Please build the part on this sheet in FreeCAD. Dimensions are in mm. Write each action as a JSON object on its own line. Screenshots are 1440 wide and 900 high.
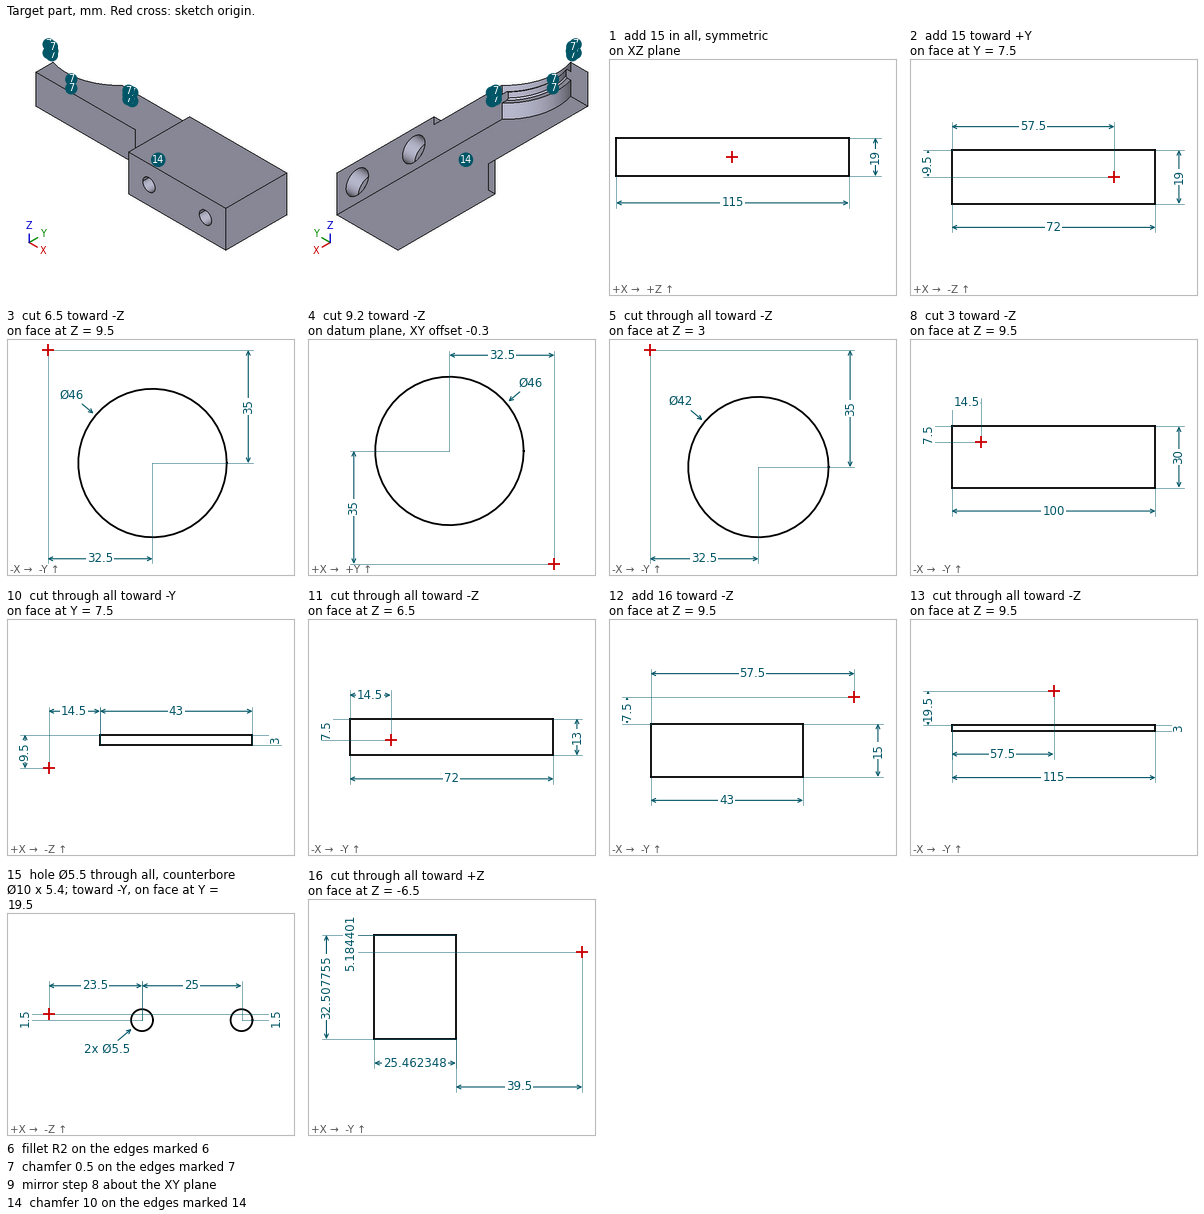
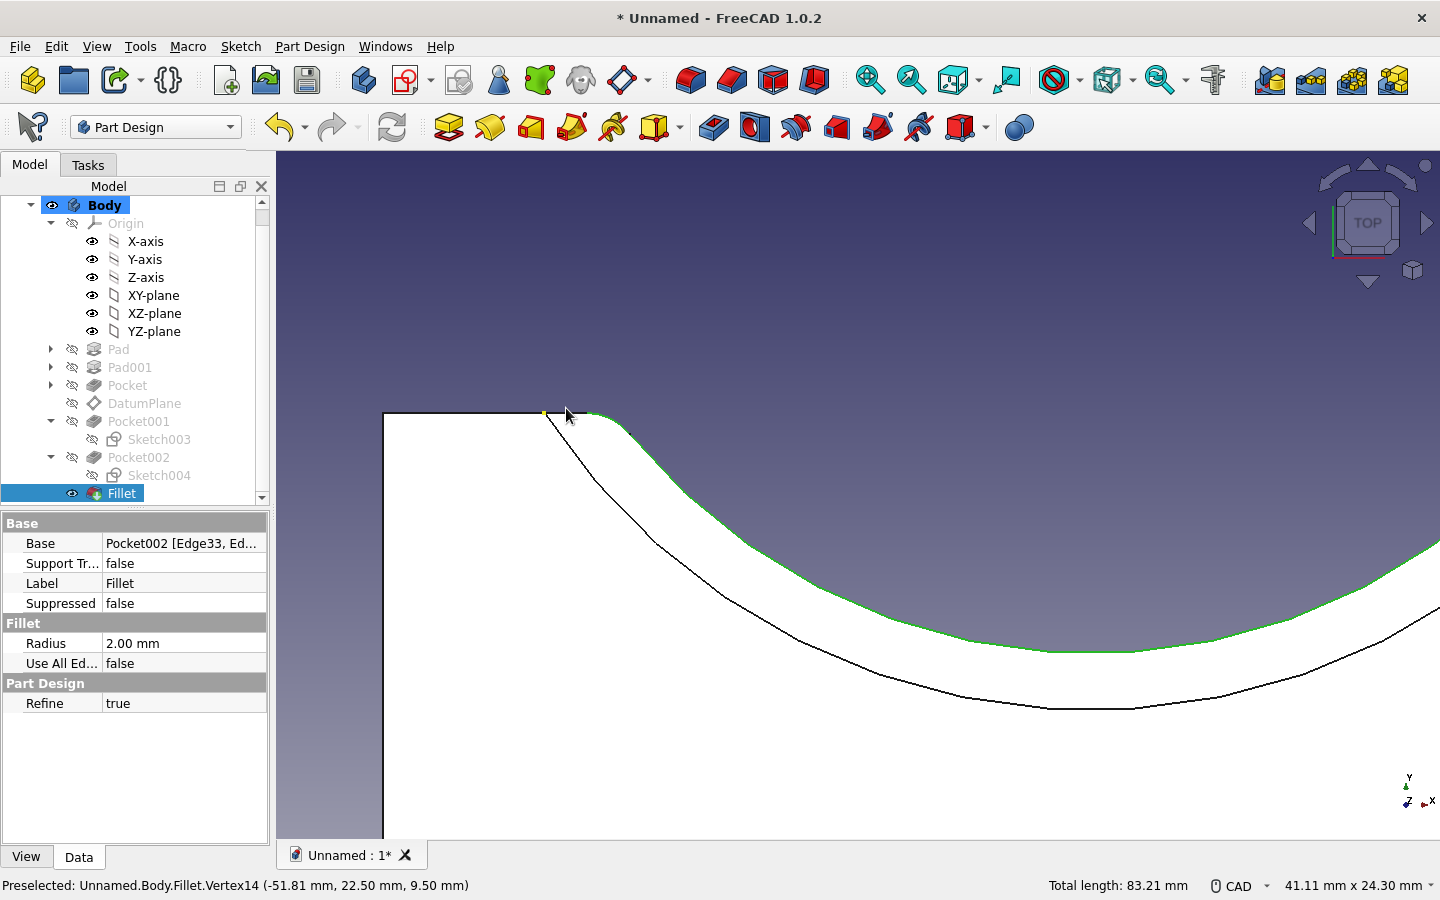
{"action": "left_click", "coordinate": [565, 412], "text": "ctrl"}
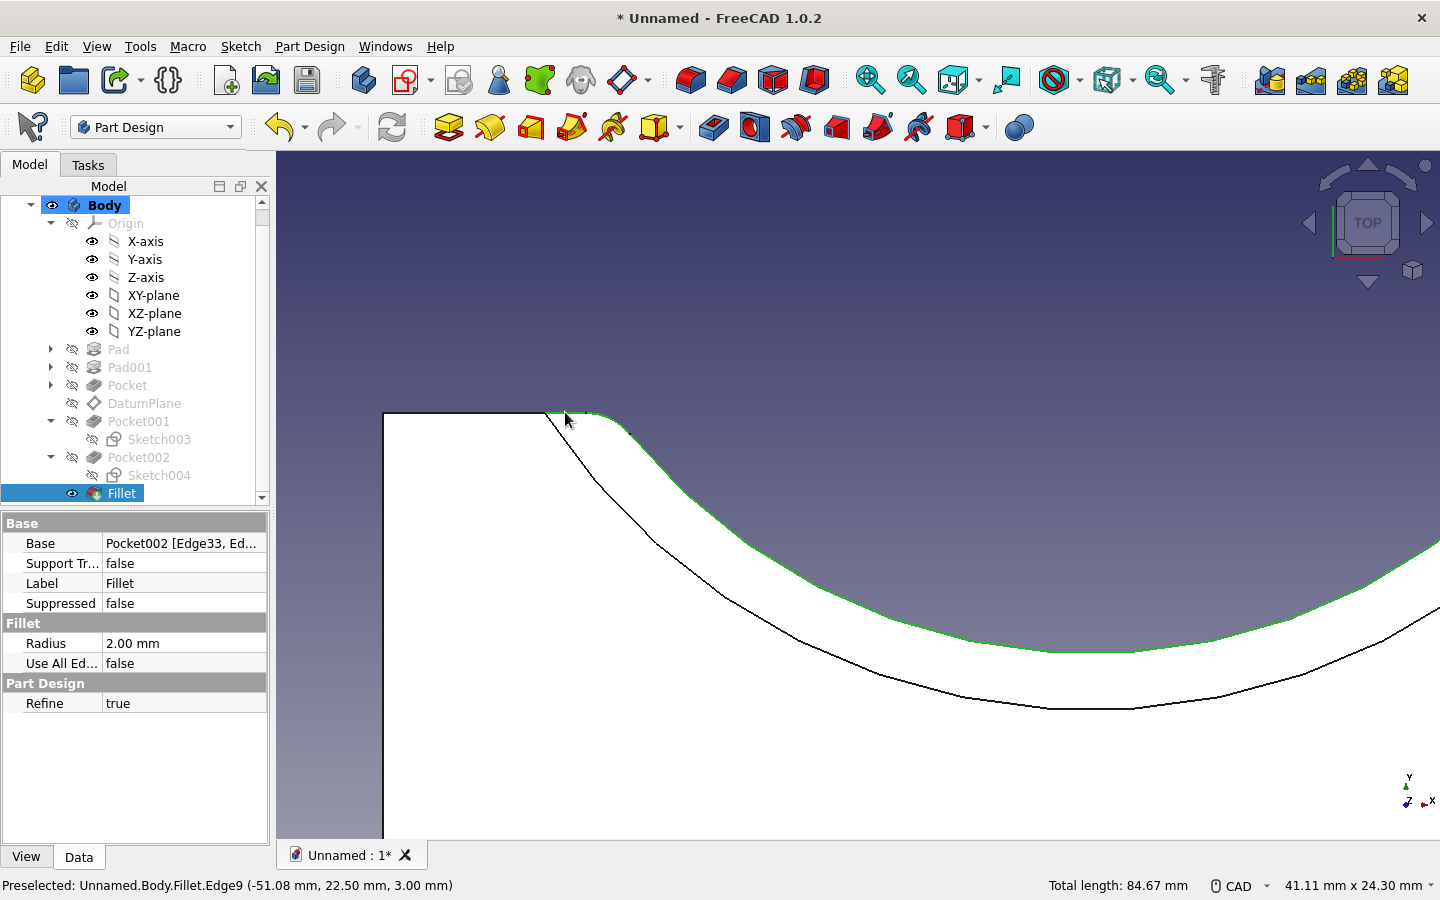
{"action": "left_click", "coordinate": [871, 80]}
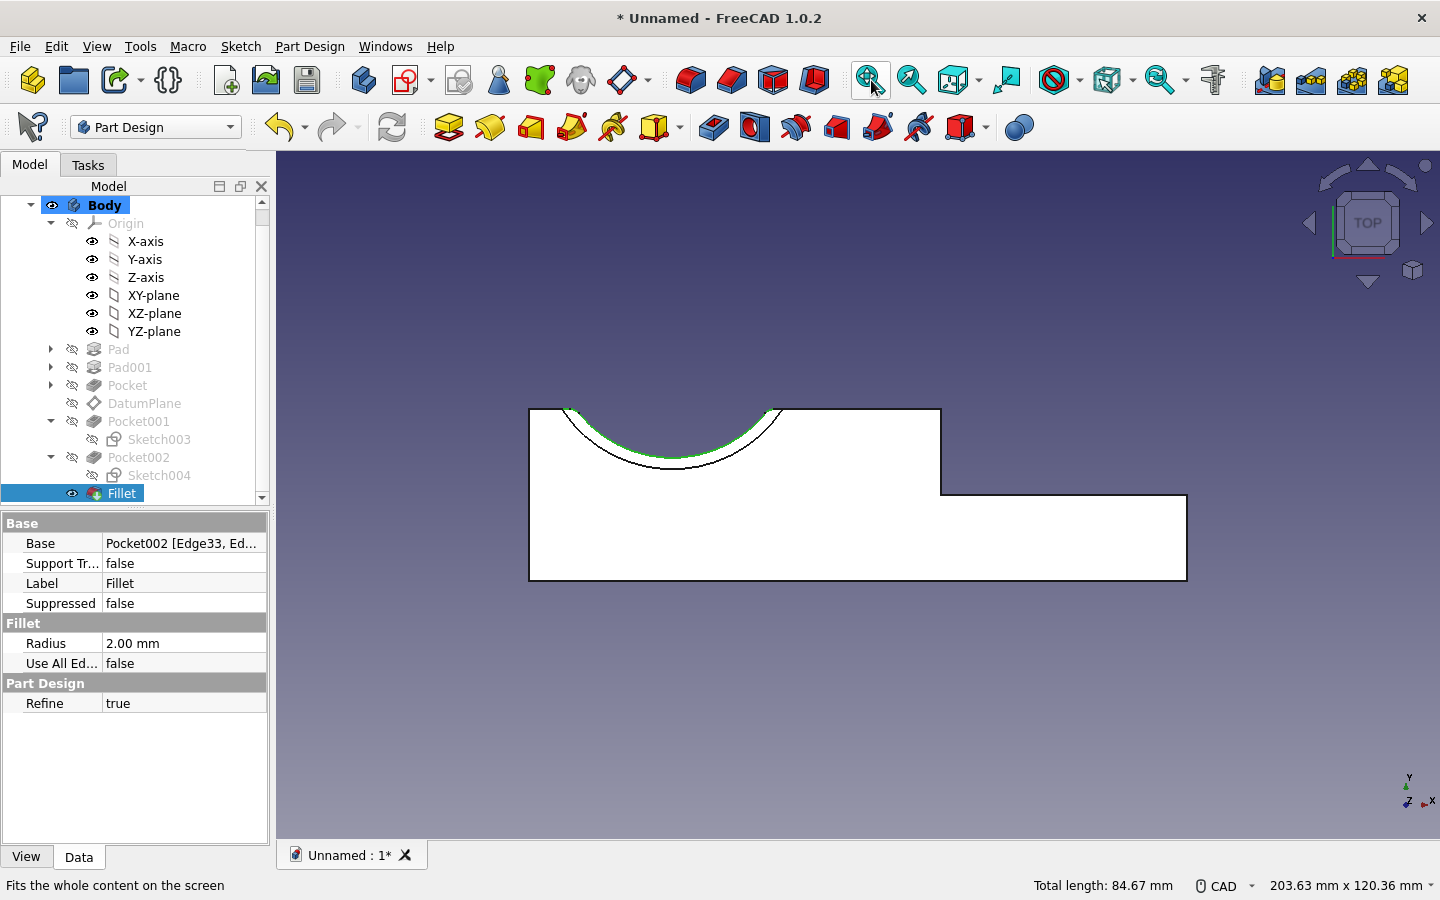
{"action": "key", "text": "1"}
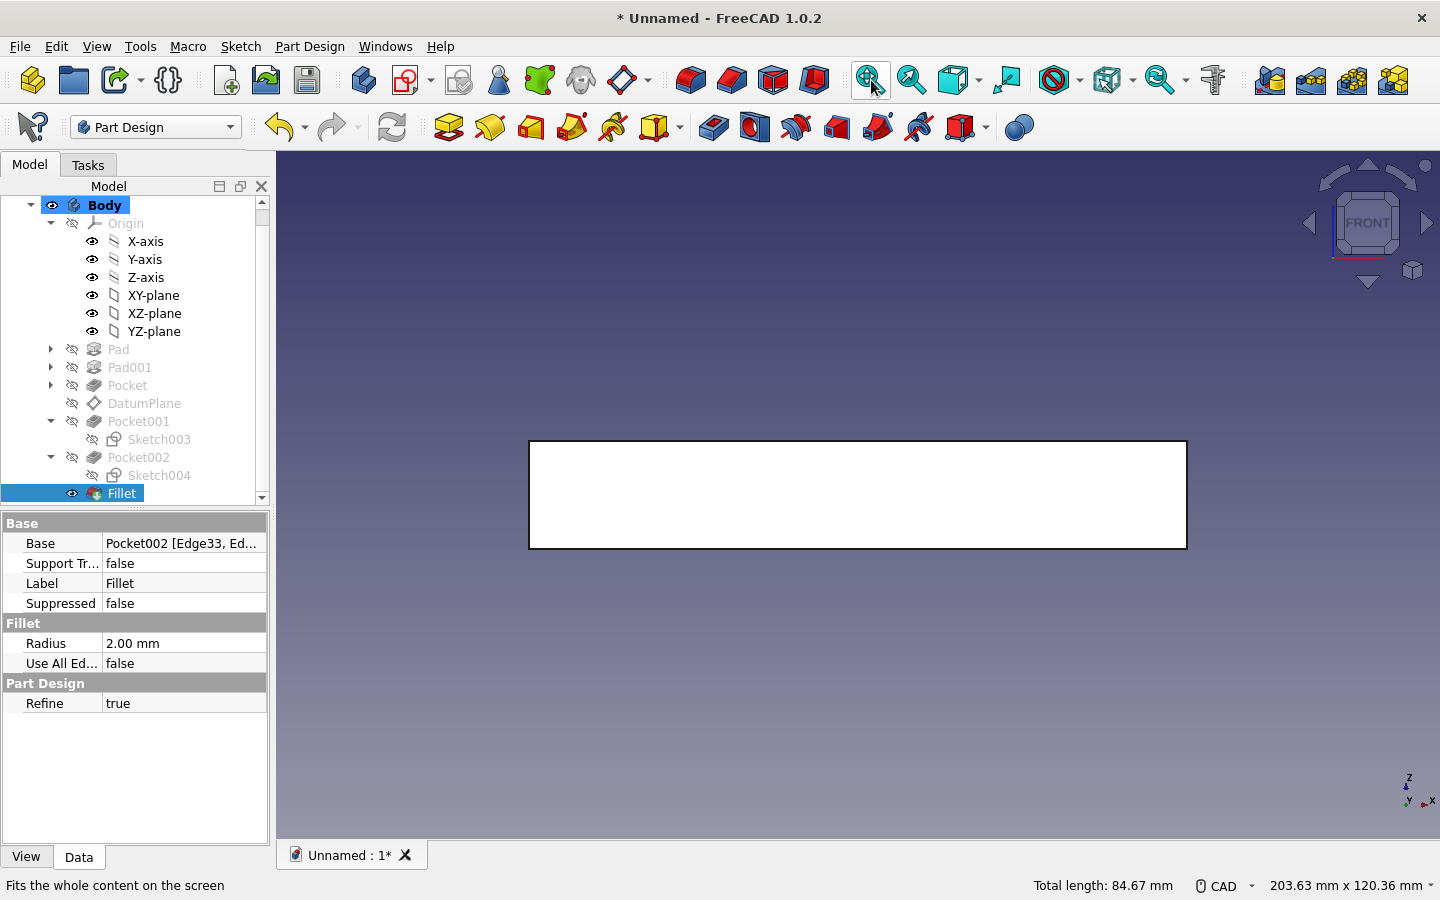
{"action": "scroll", "coordinate": [778, 496], "scroll_direction": "up", "scroll_amount": 8}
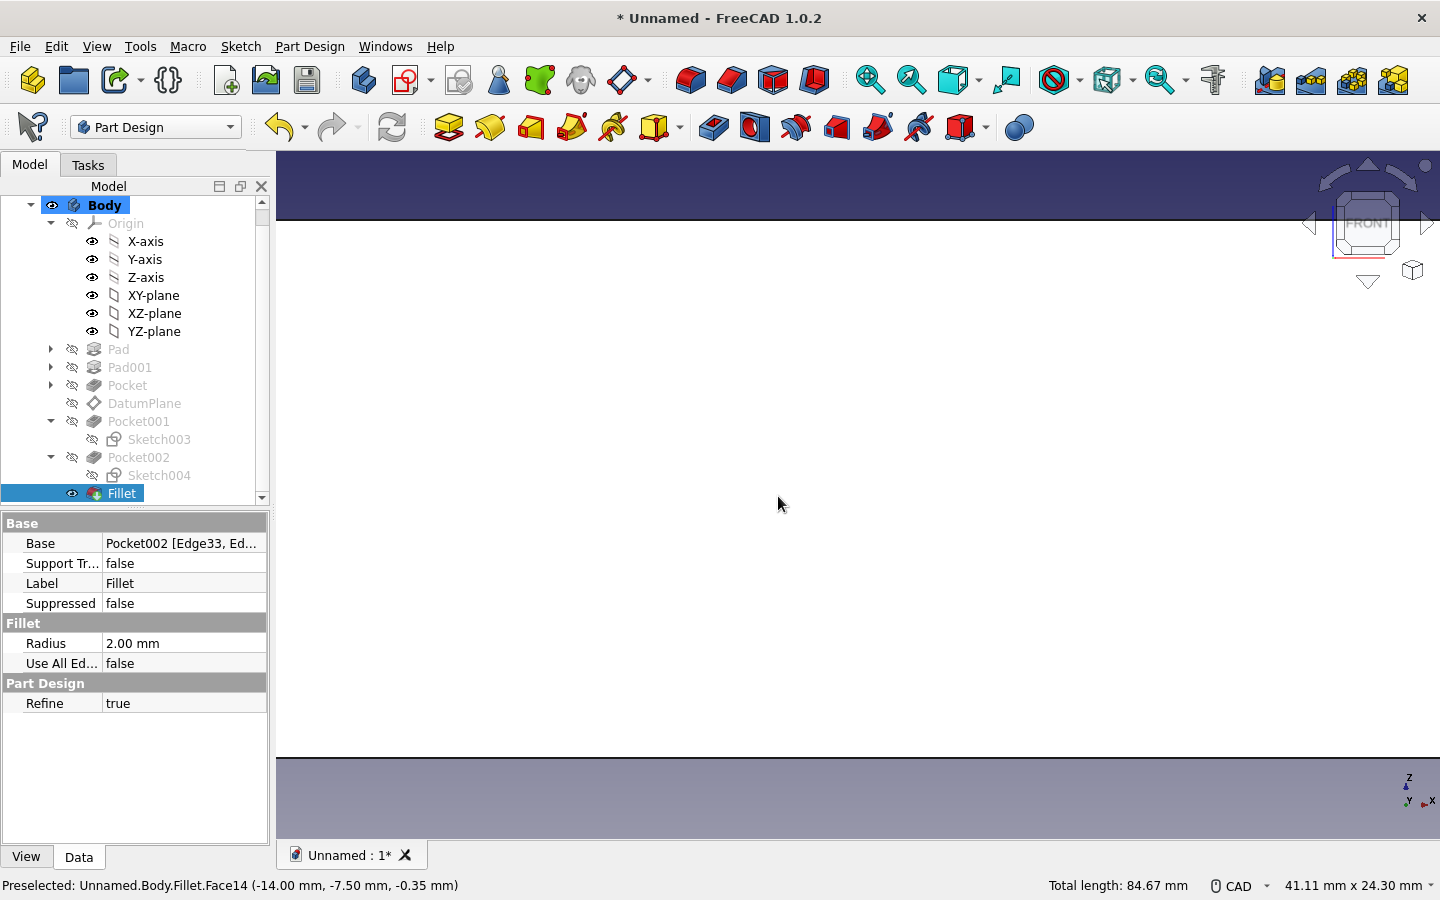
{"action": "left_click", "coordinate": [871, 80]}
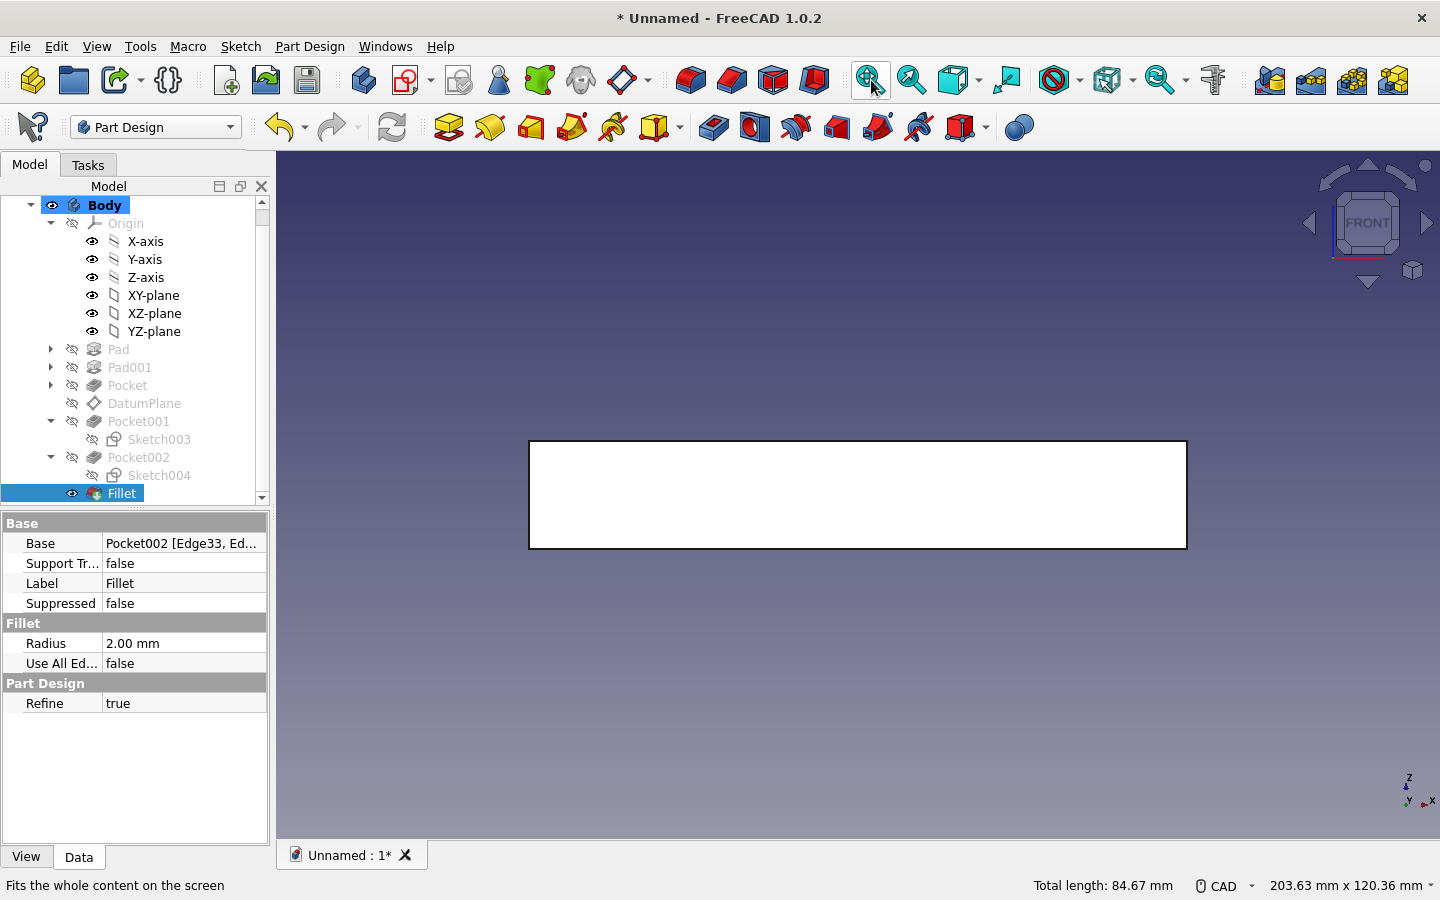
{"action": "key", "text": "3"}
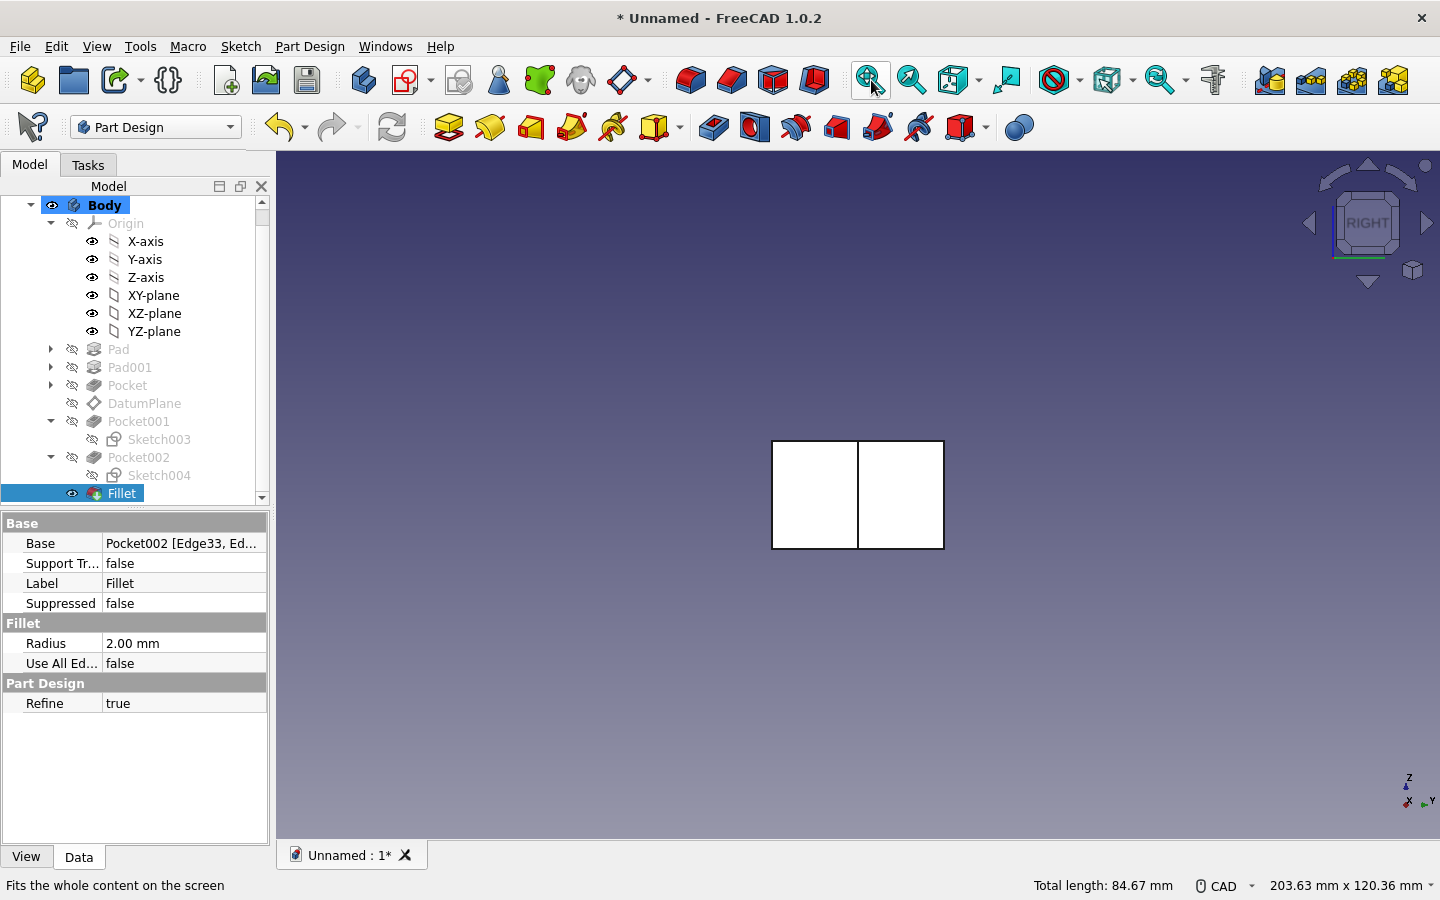
{"action": "left_click", "coordinate": [871, 80]}